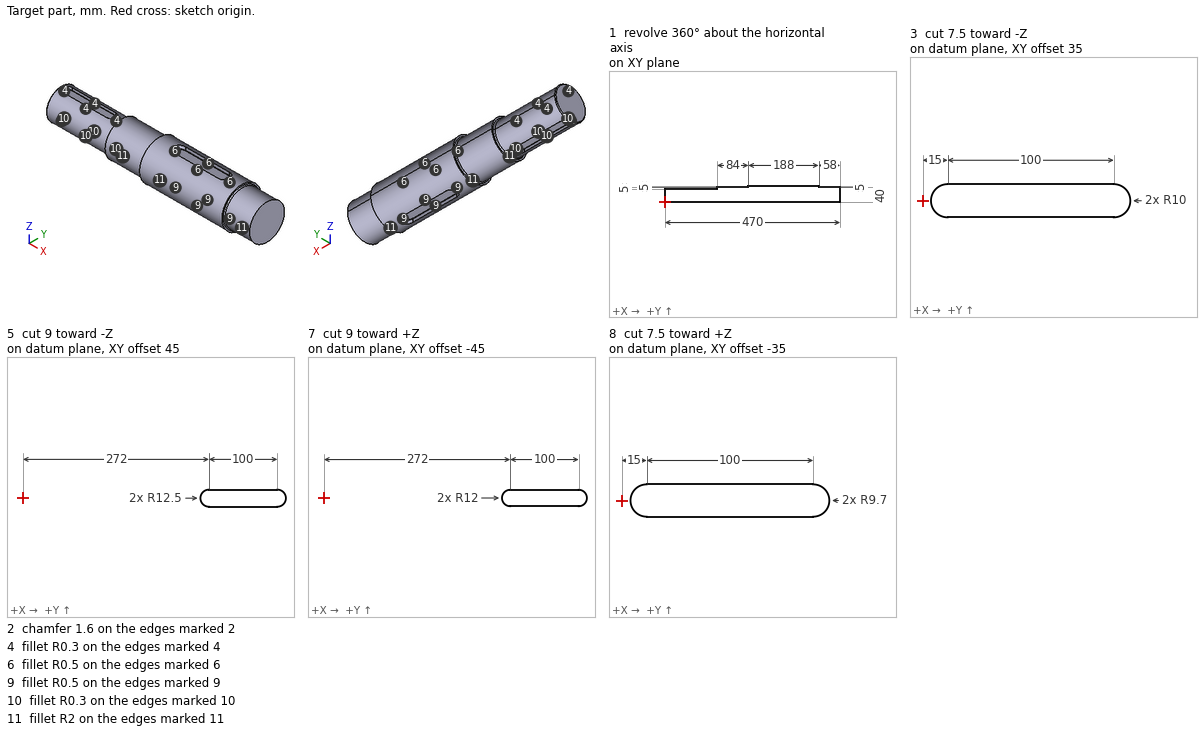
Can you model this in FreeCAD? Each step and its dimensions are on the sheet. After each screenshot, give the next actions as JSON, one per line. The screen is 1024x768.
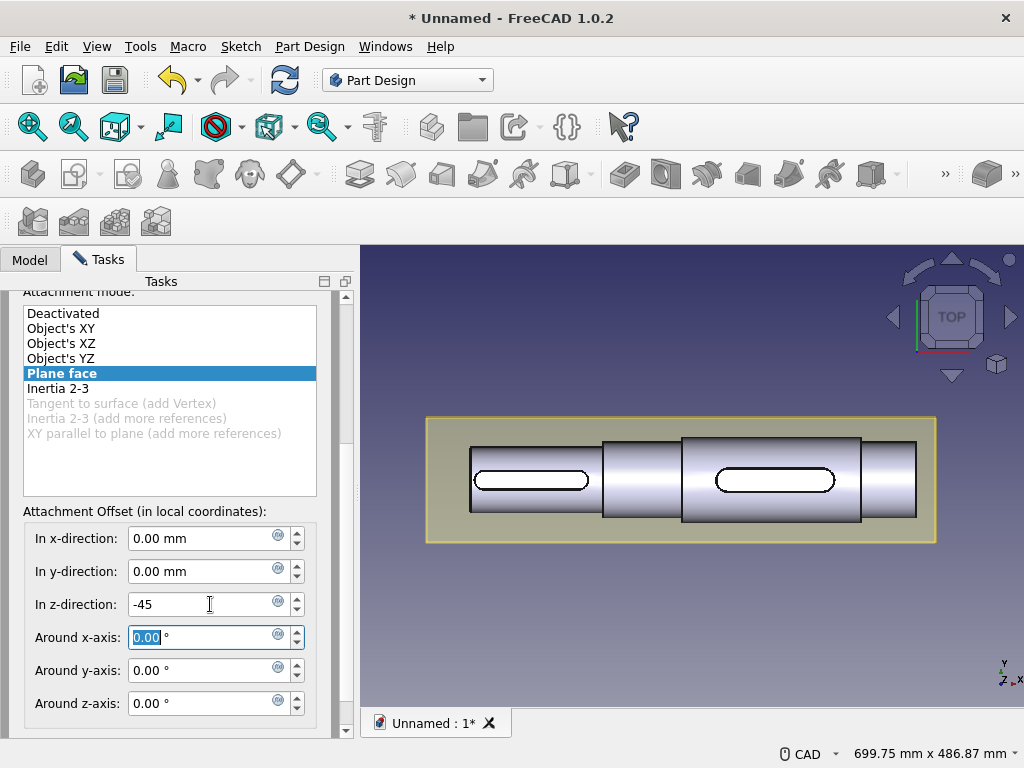
{"action": "scroll", "coordinate": [346, 514], "scroll_direction": "up", "scroll_amount": 5}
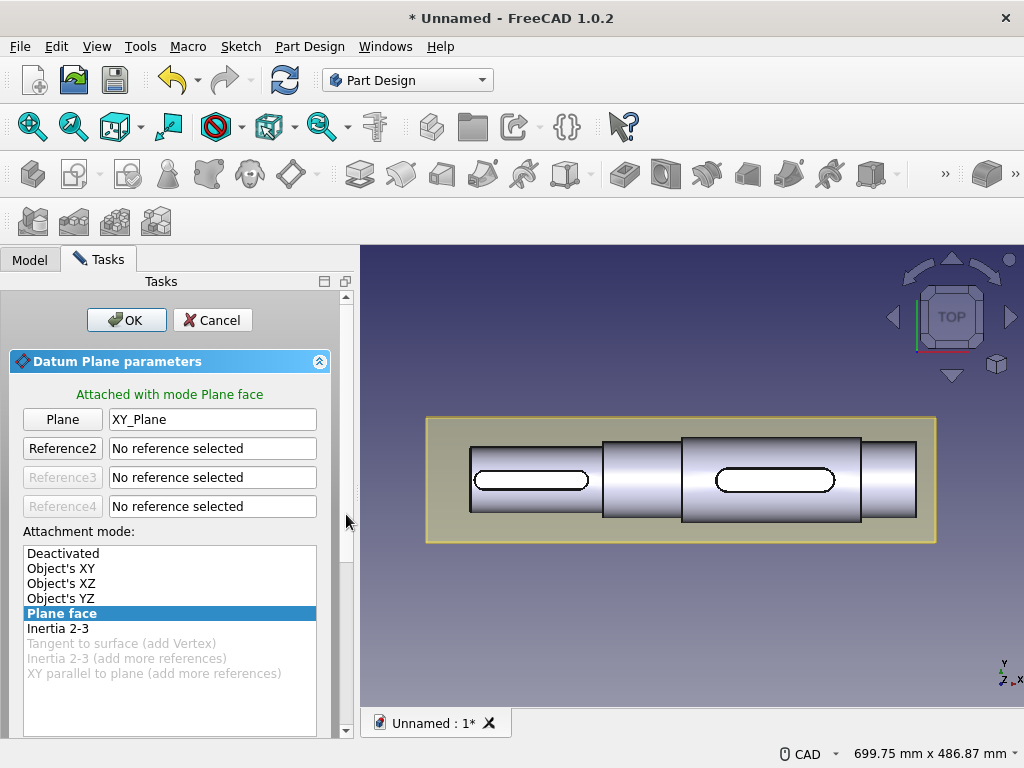
{"action": "left_click", "coordinate": [127, 320]}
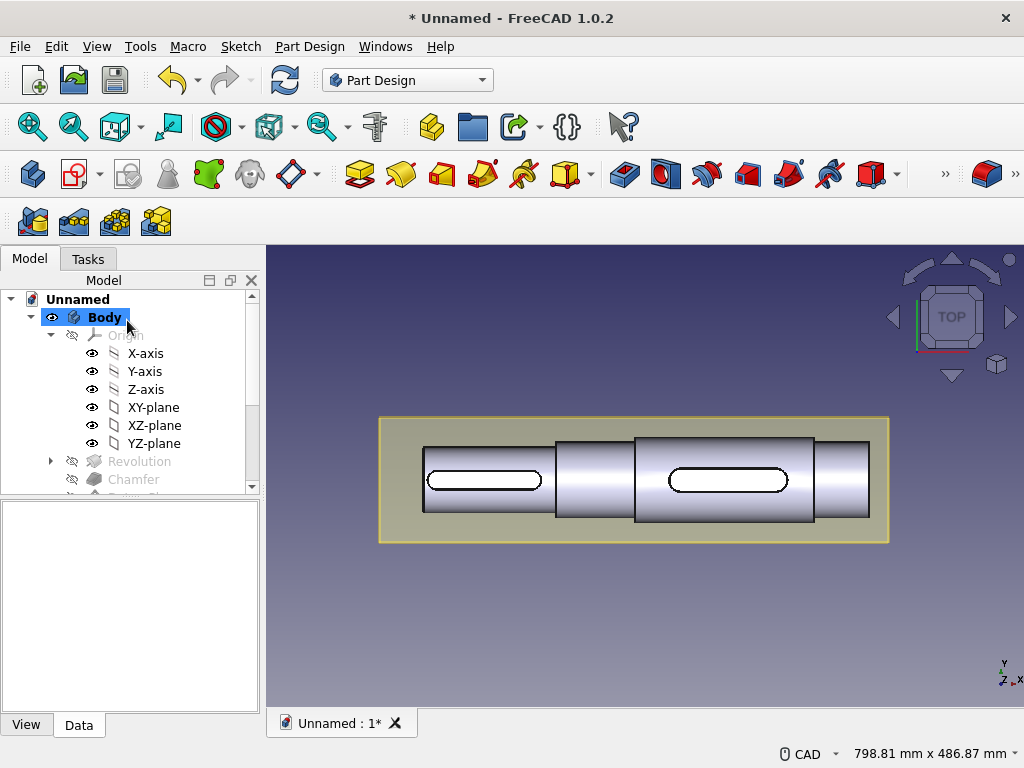
{"action": "scroll", "coordinate": [101, 385], "scroll_direction": "down", "scroll_amount": 3}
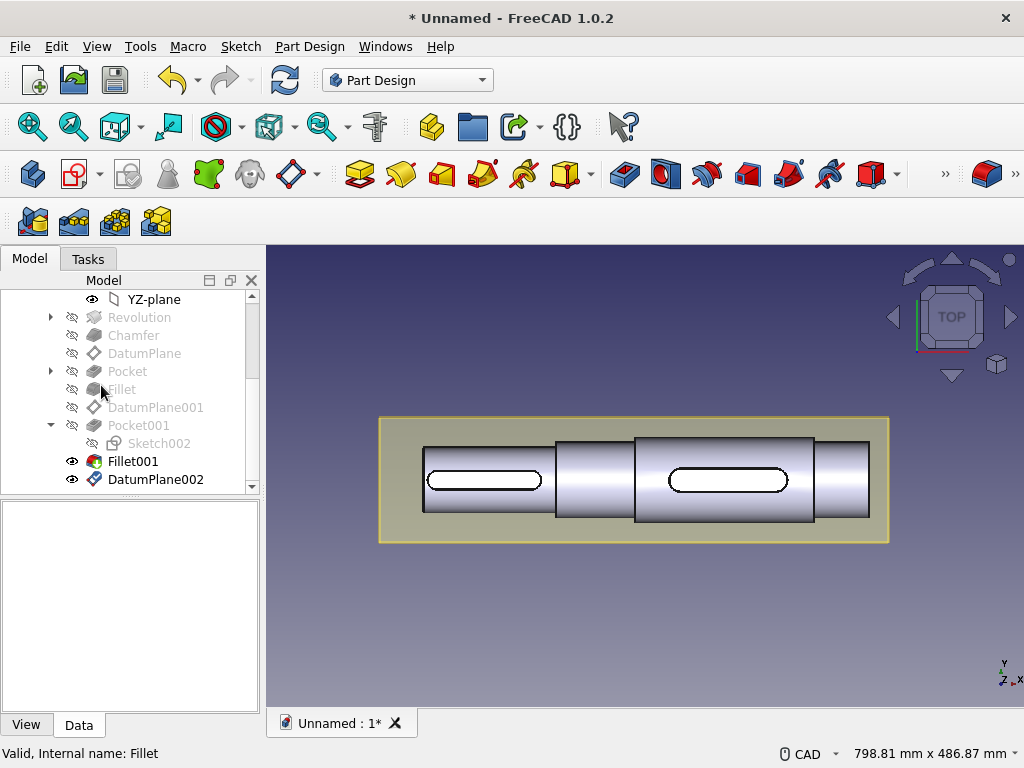
{"action": "left_click", "coordinate": [117, 479]}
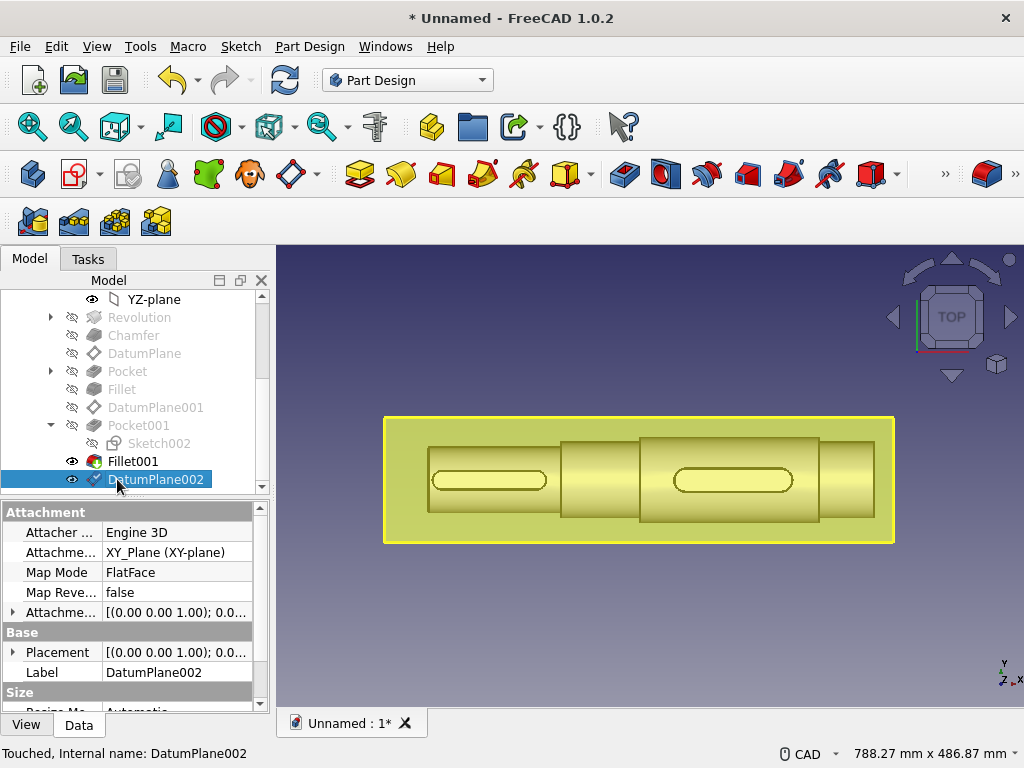
{"action": "left_click", "coordinate": [74, 174]}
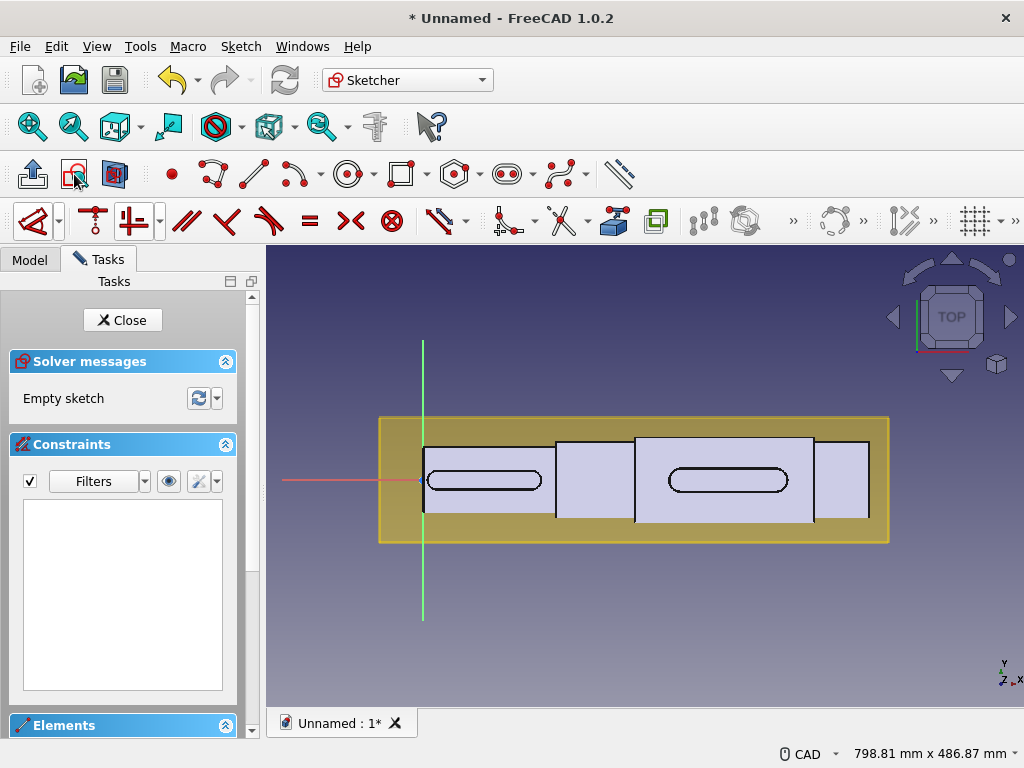
{"action": "left_click", "coordinate": [115, 174]}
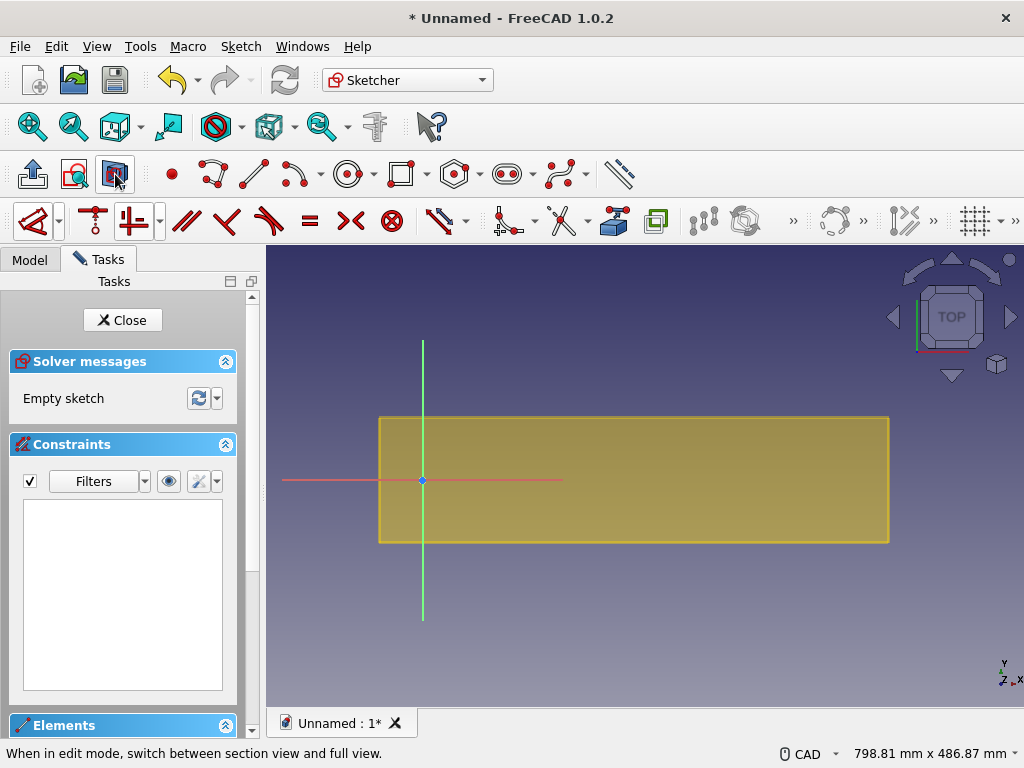
{"action": "scroll", "coordinate": [794, 482], "scroll_direction": "up", "scroll_amount": 6}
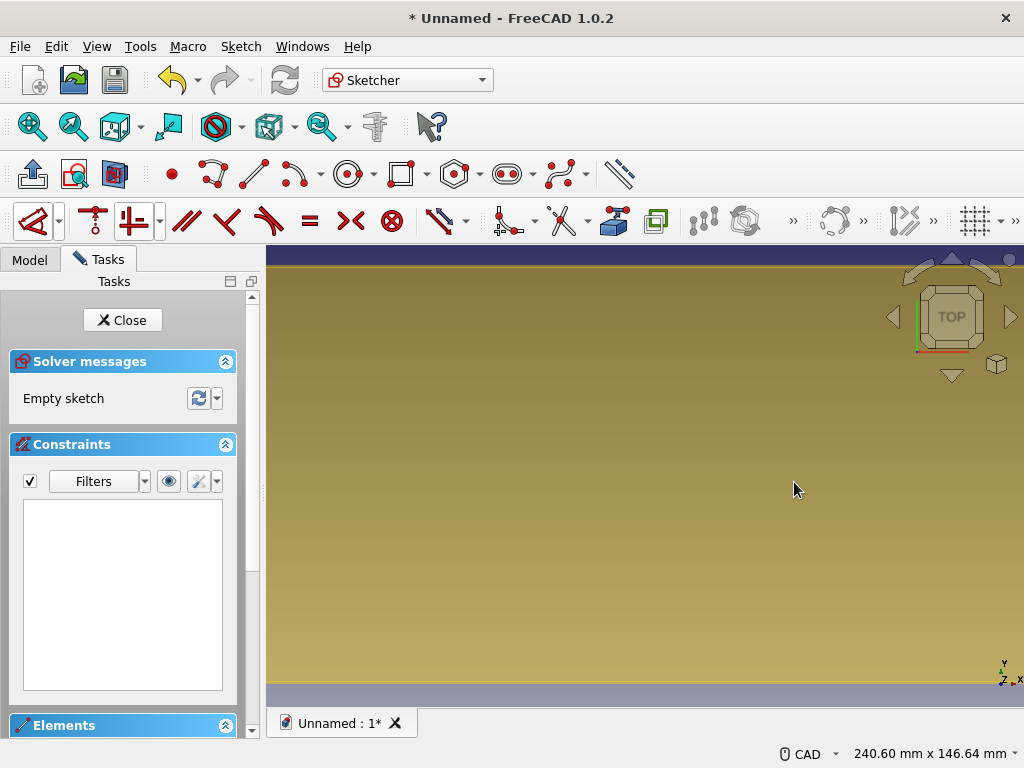
{"action": "left_click", "coordinate": [506, 174]}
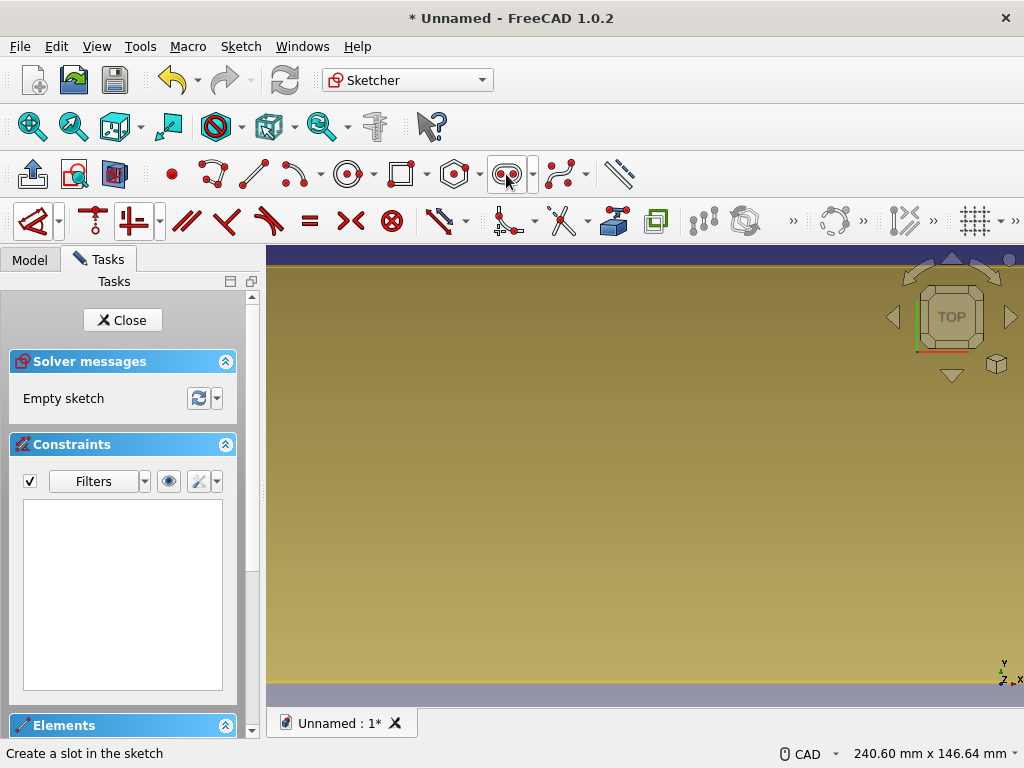
{"action": "left_click", "coordinate": [417, 475]}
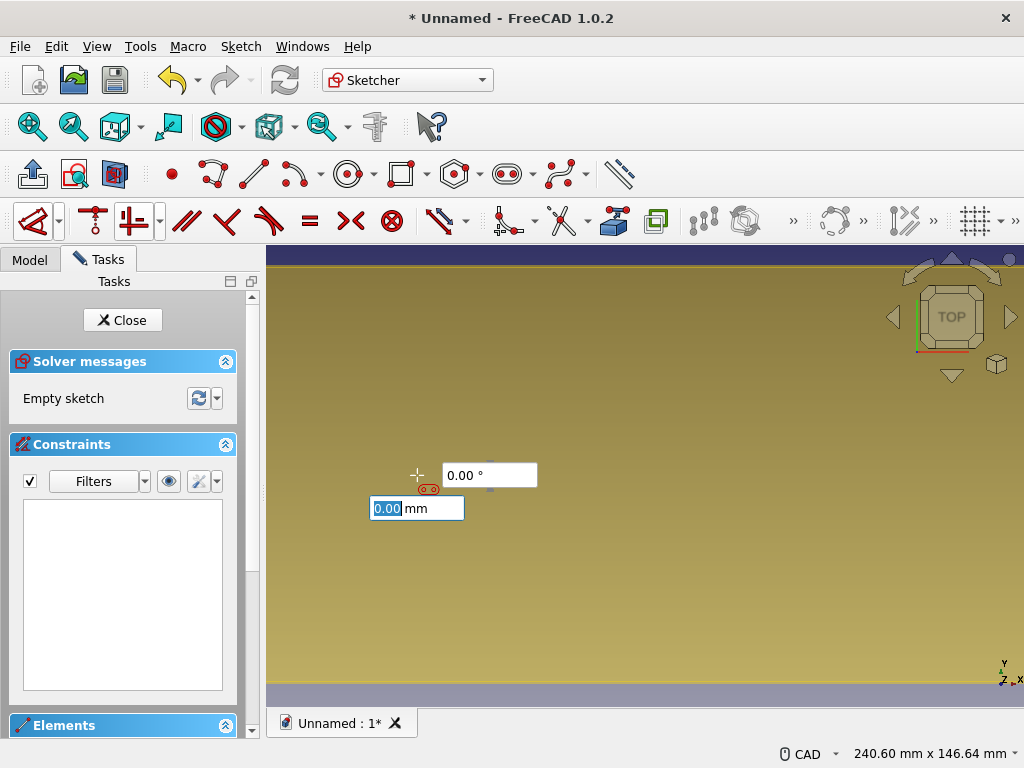
{"action": "left_click", "coordinate": [732, 466]}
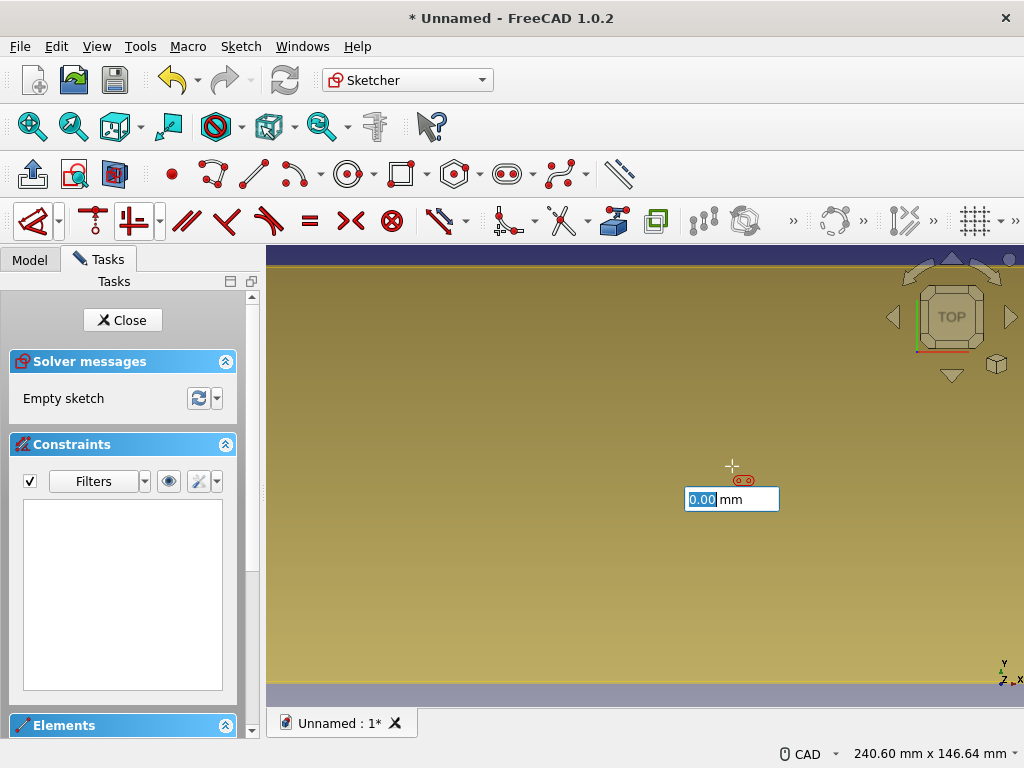
{"action": "left_click", "coordinate": [574, 437]}
{"action": "key", "text": "Escape"}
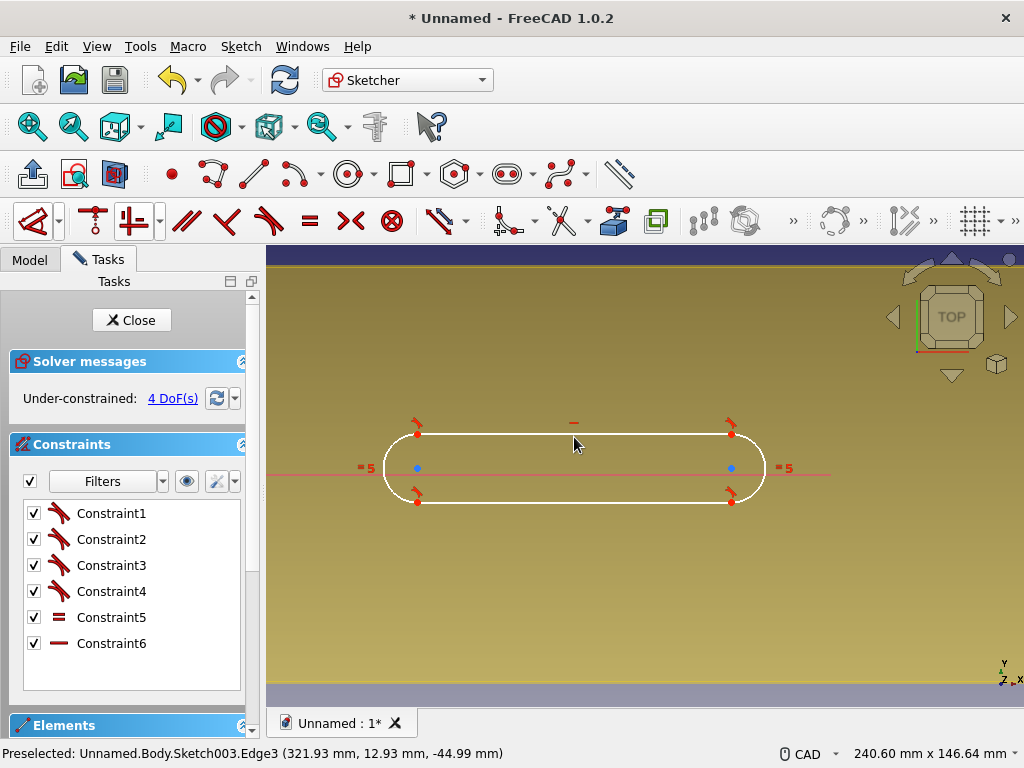
{"action": "left_click", "coordinate": [418, 468]}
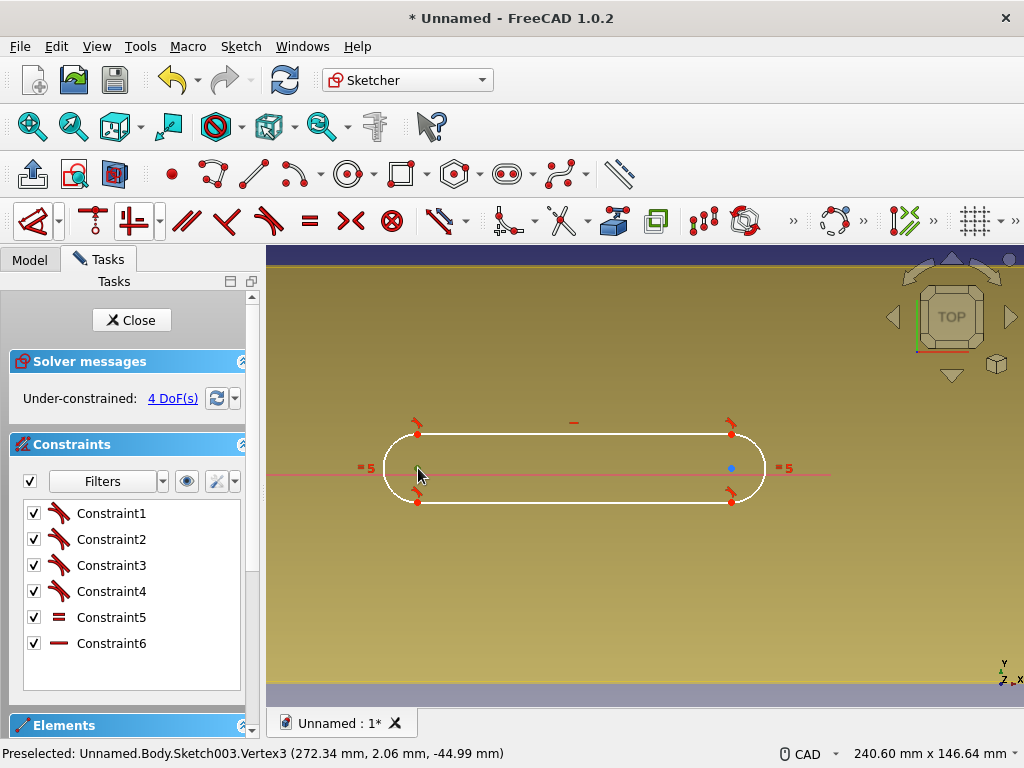
{"action": "left_click", "coordinate": [334, 475]}